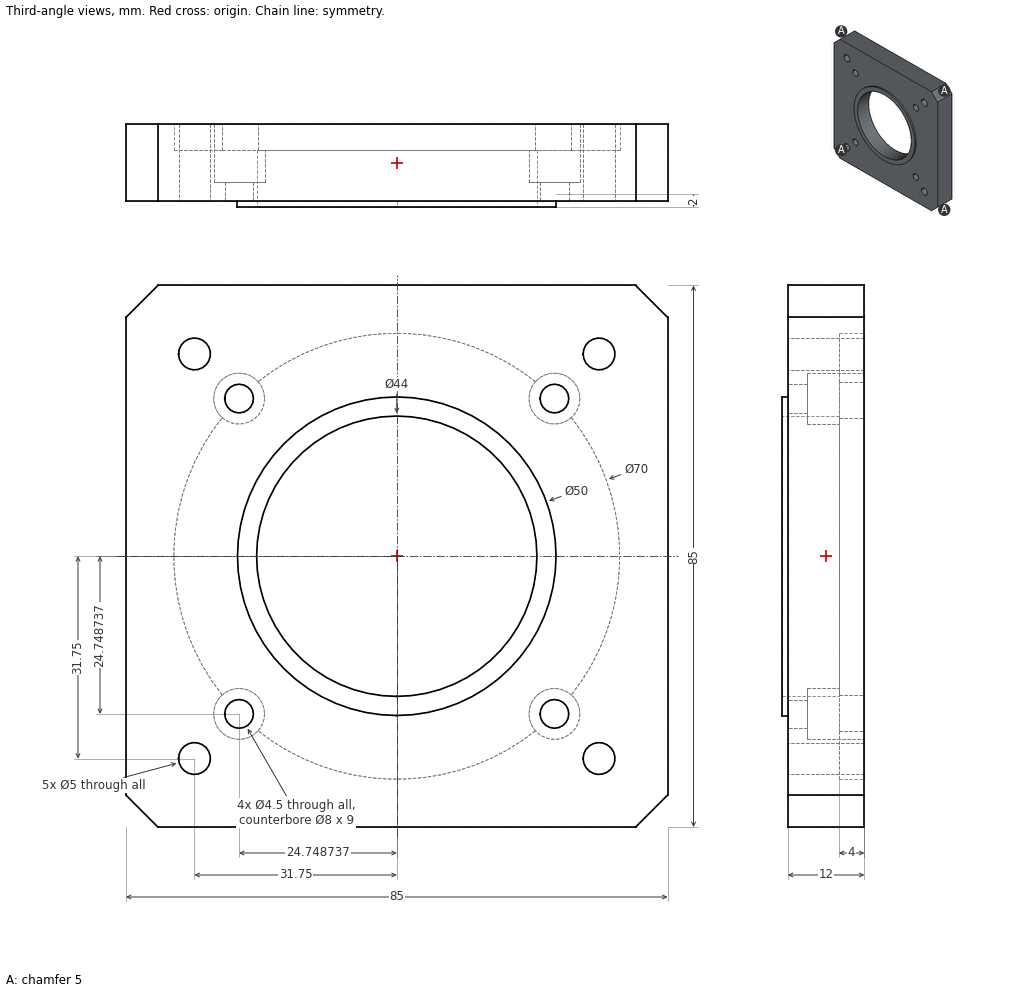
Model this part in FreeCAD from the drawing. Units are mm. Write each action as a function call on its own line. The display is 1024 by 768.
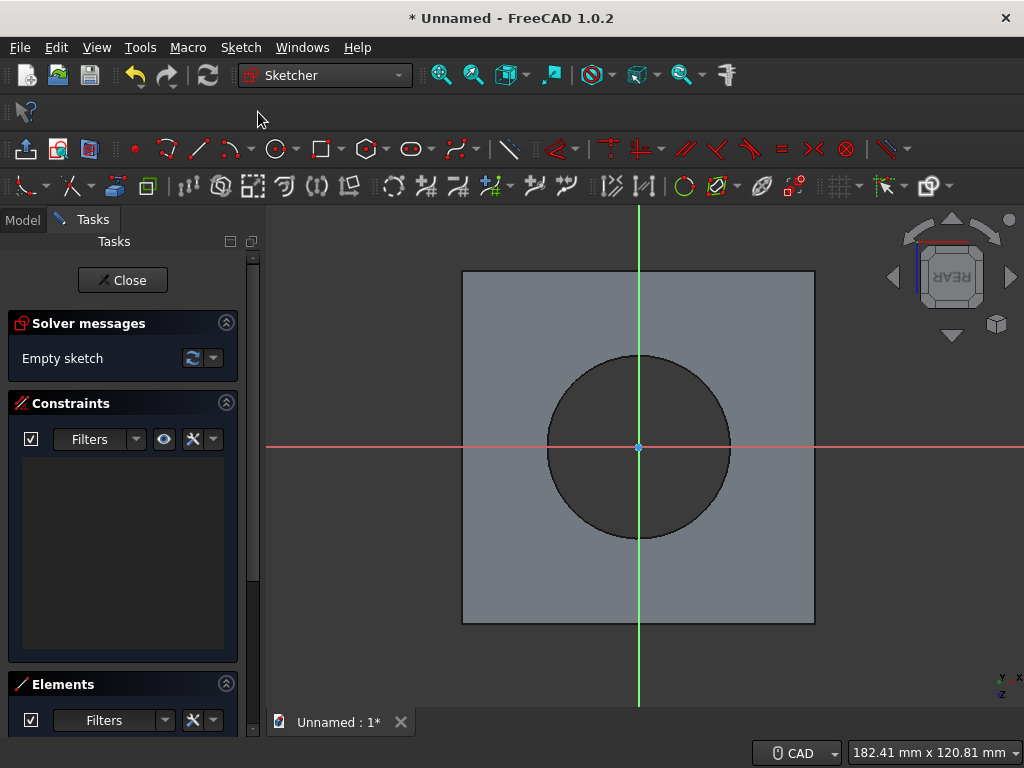
click(276, 150)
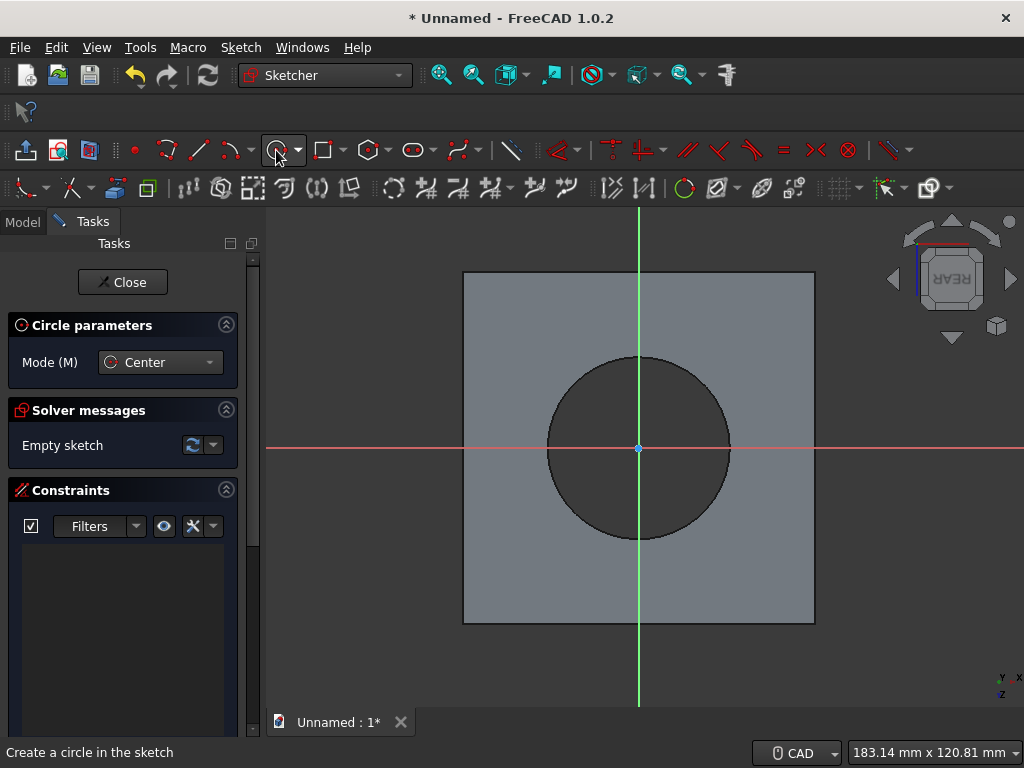
click(639, 448)
move(741, 346)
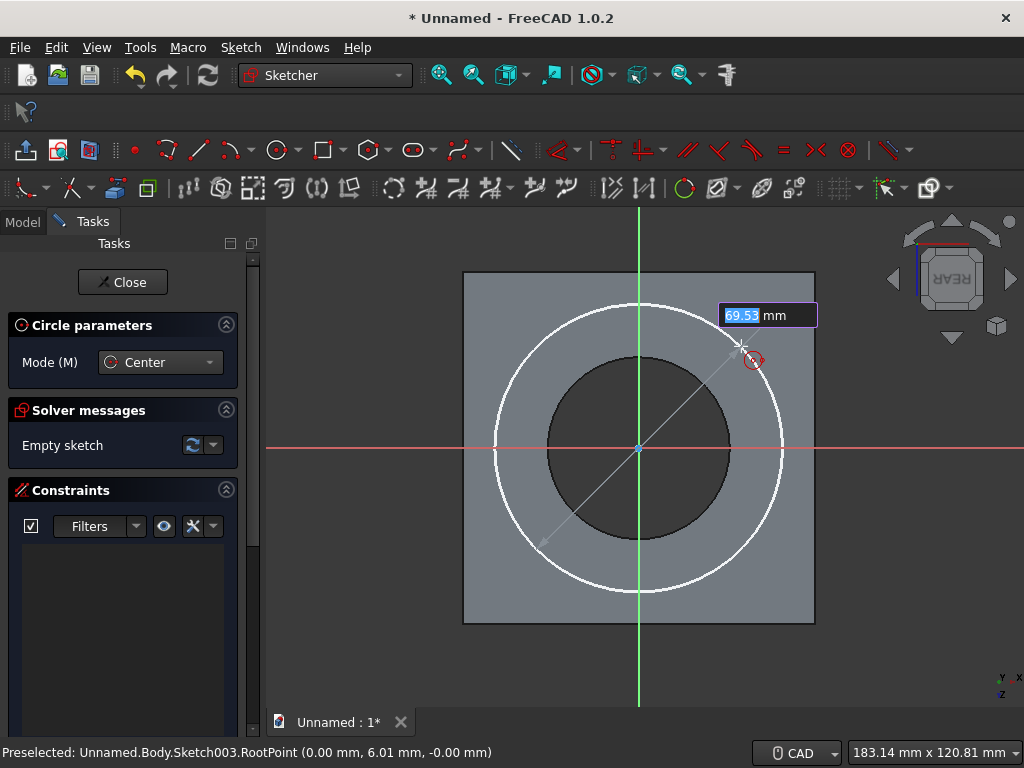
text(70)
key(Return)
key(Escape)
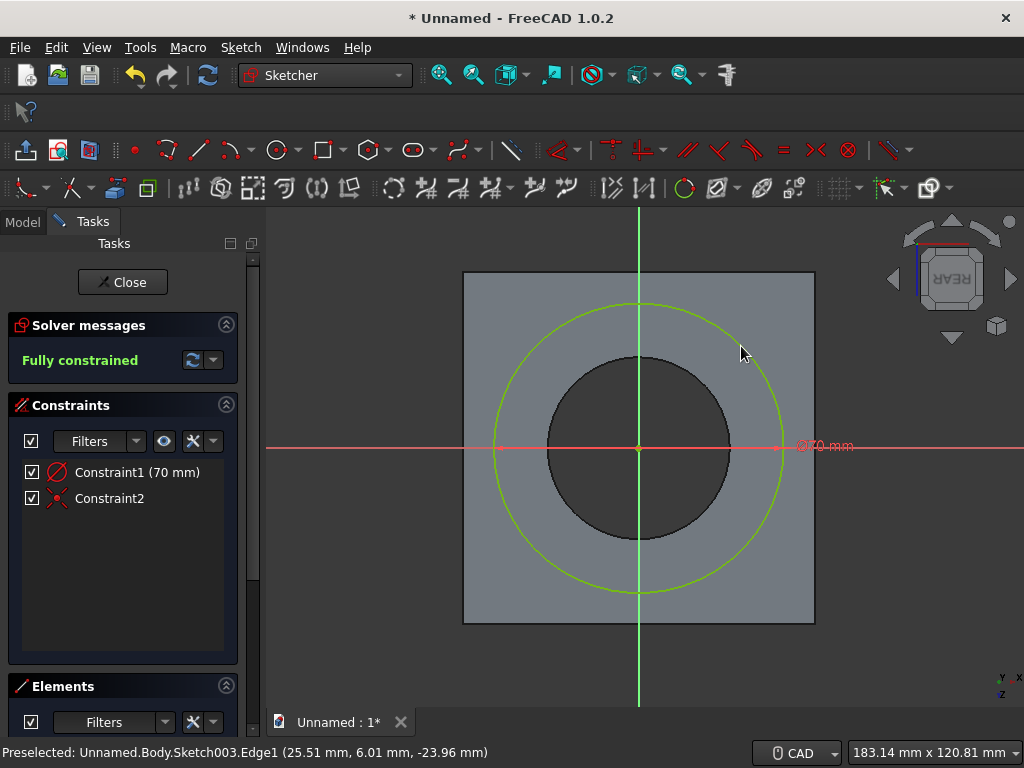
click(123, 282)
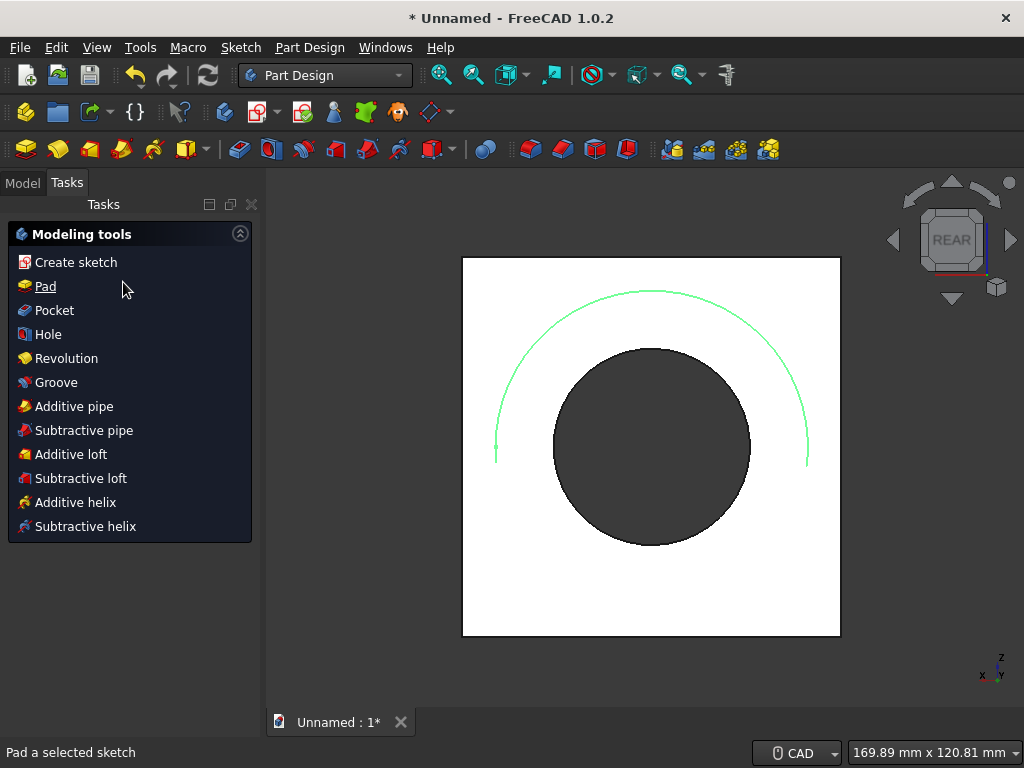
click(240, 150)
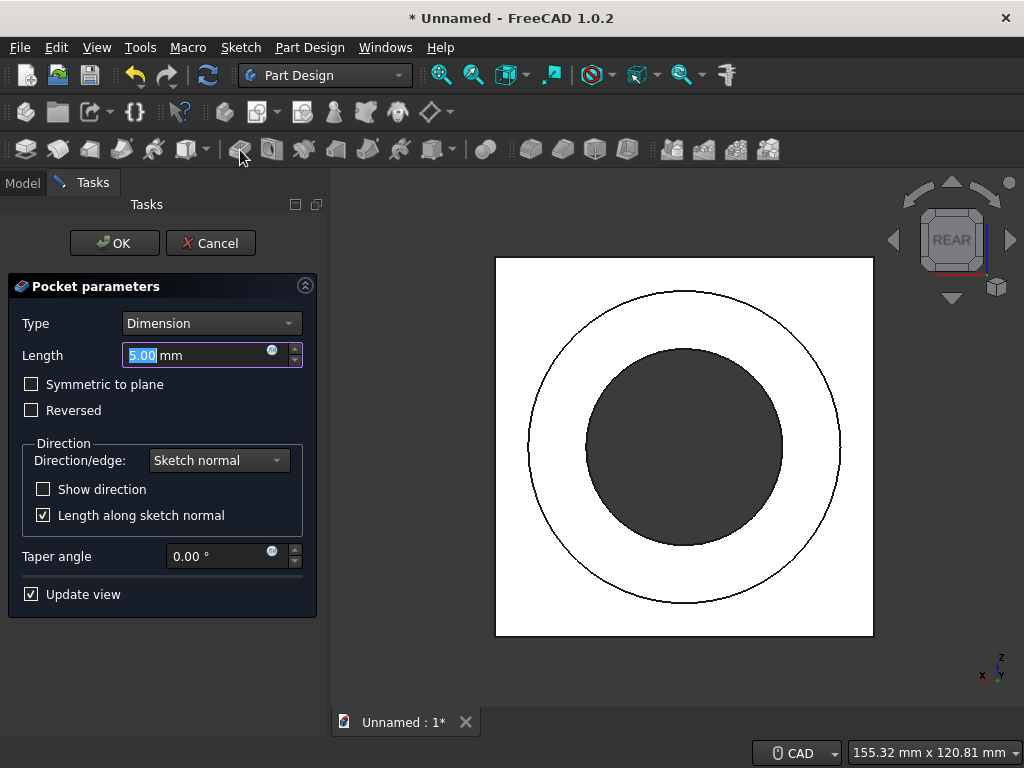
text(4)
key(Tab)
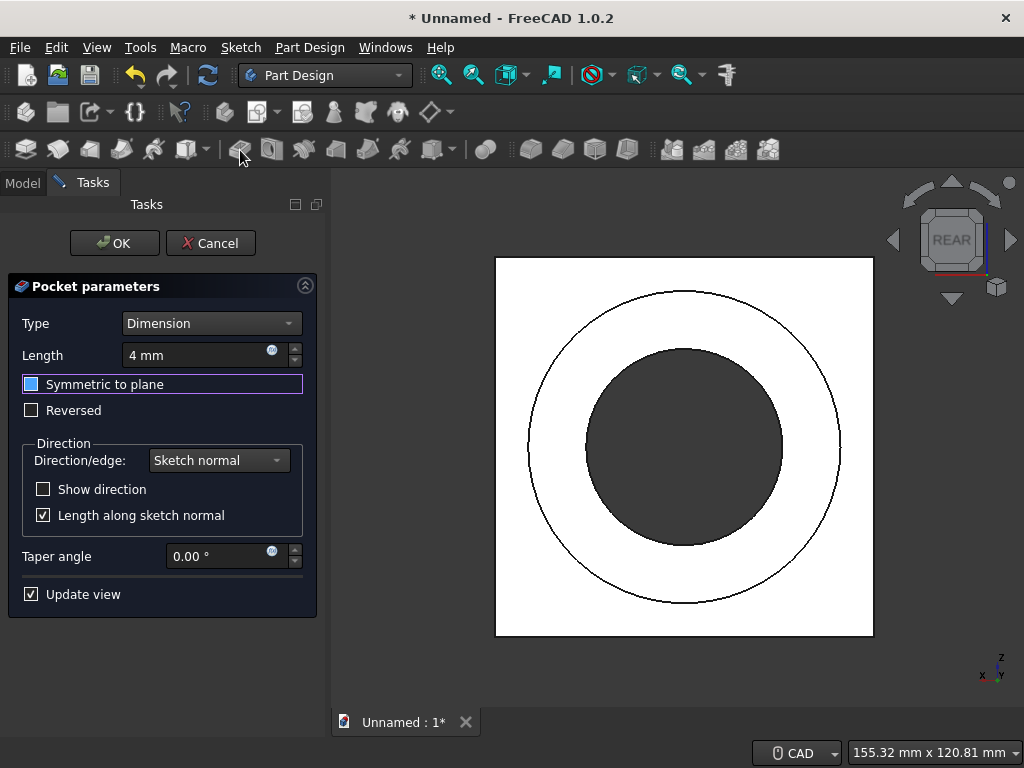
click(115, 243)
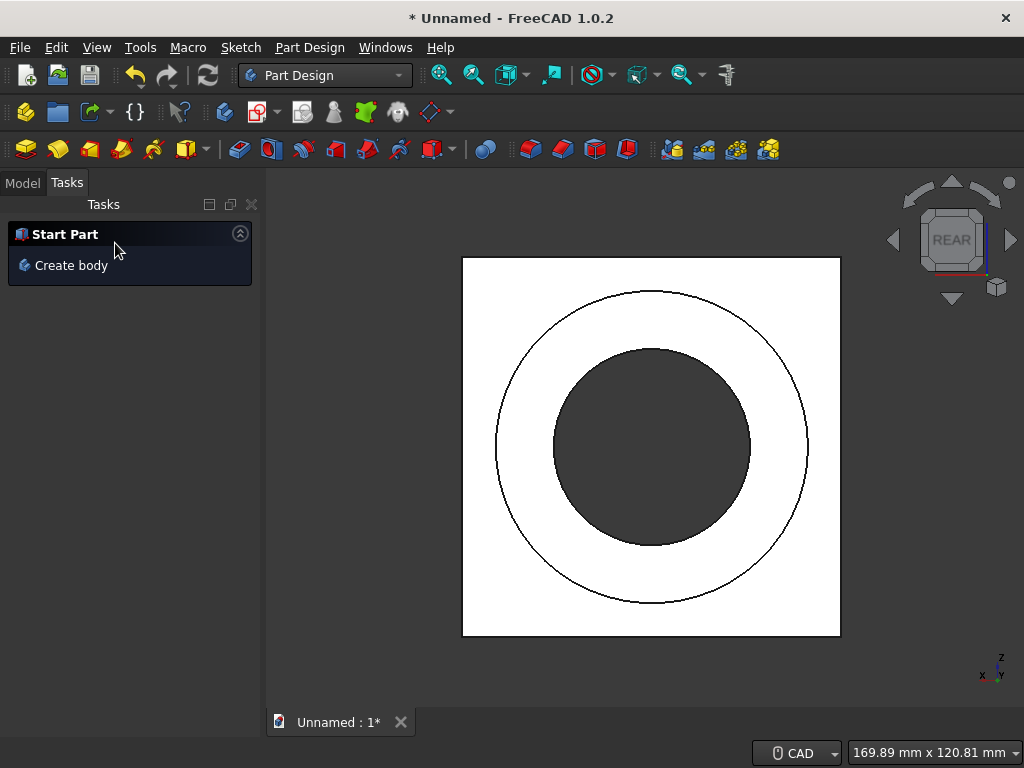
click(489, 284)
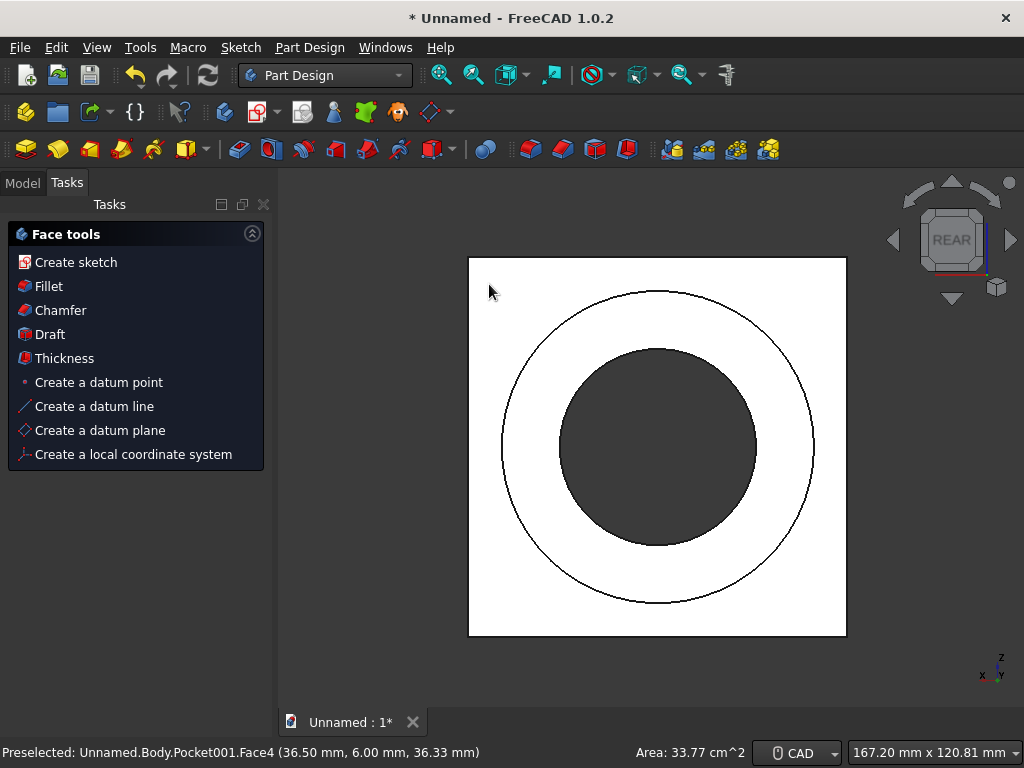
click(258, 112)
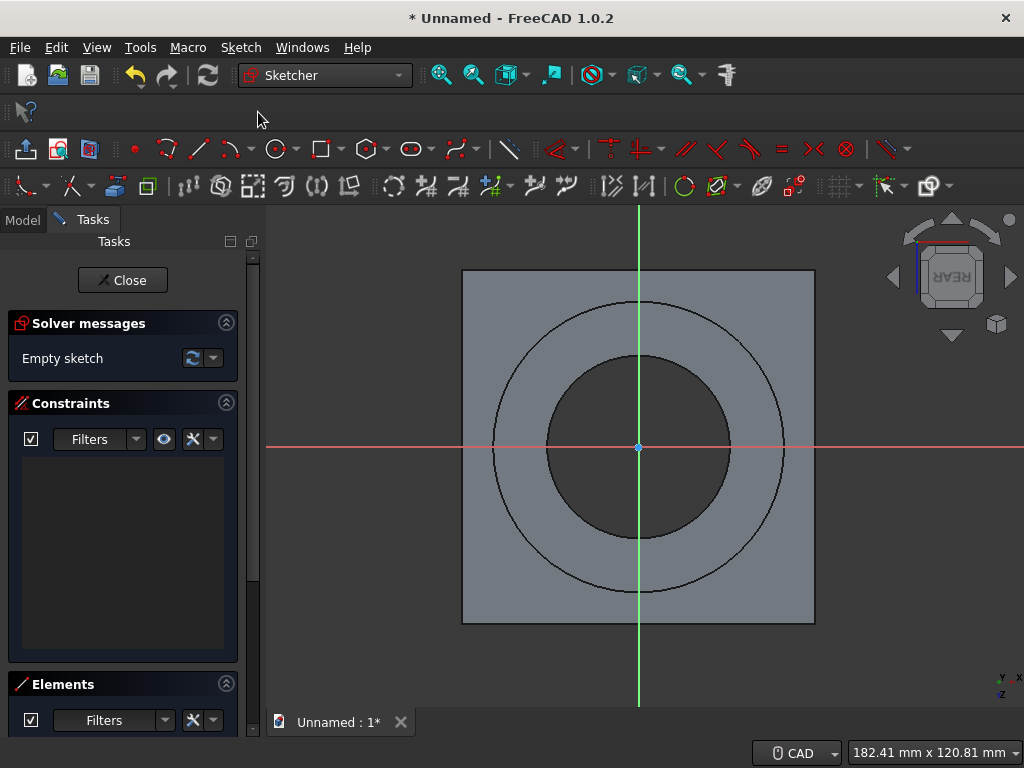
click(276, 150)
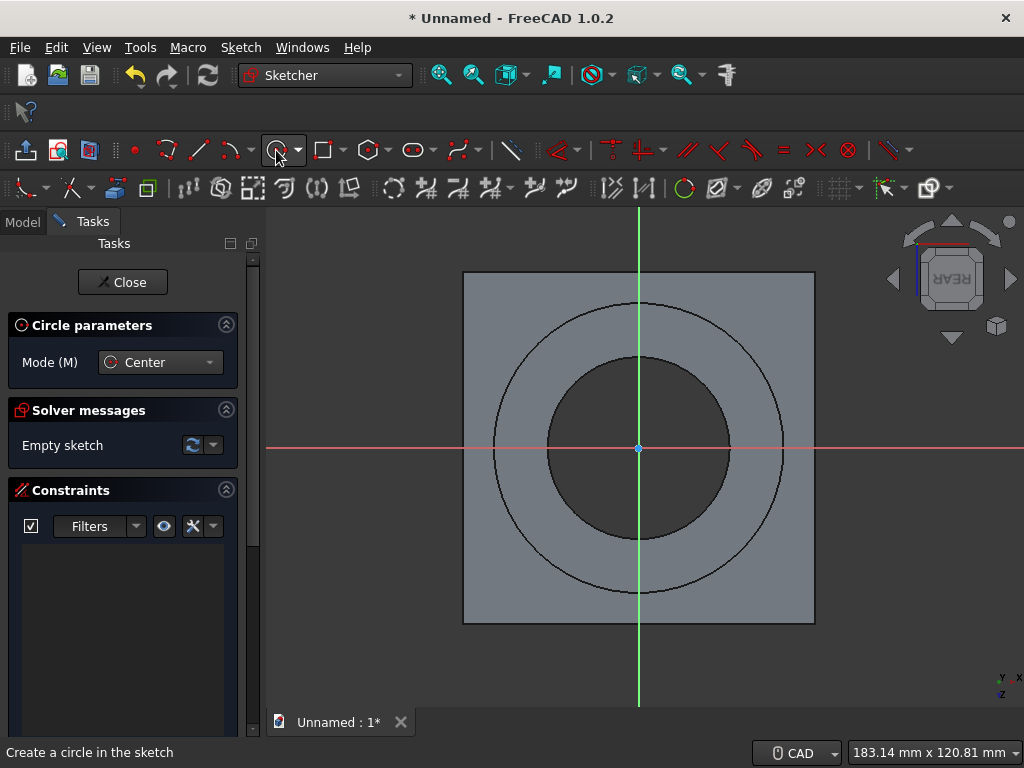
scroll(507, 317, up, 4)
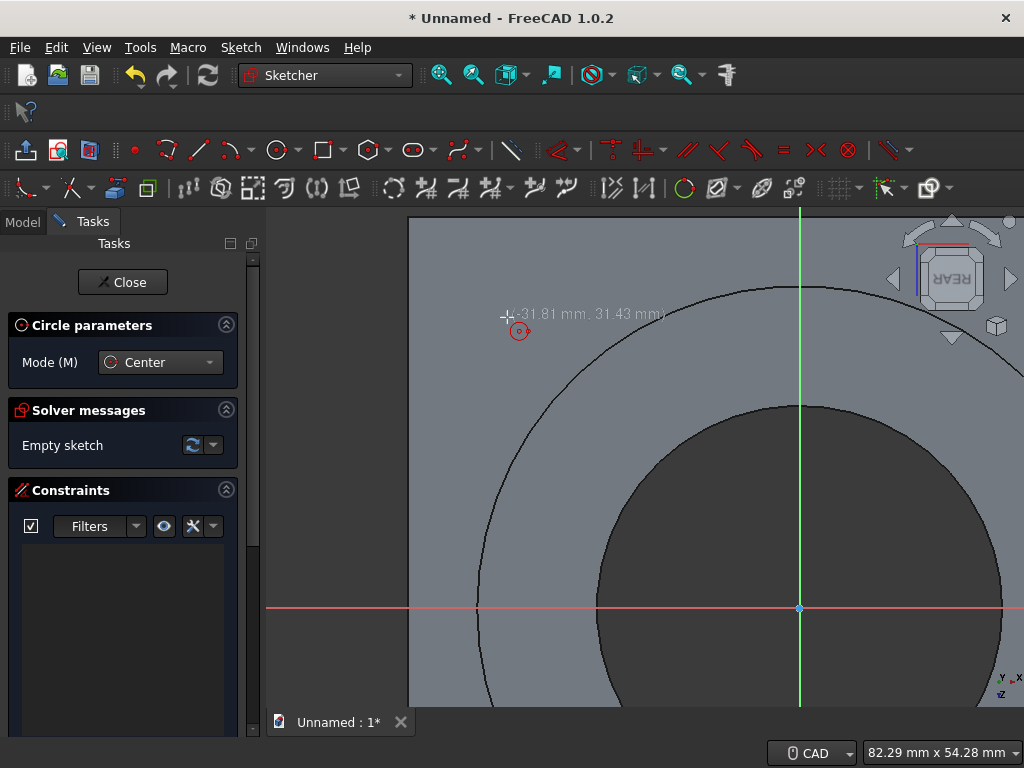
click(507, 316)
move(523, 300)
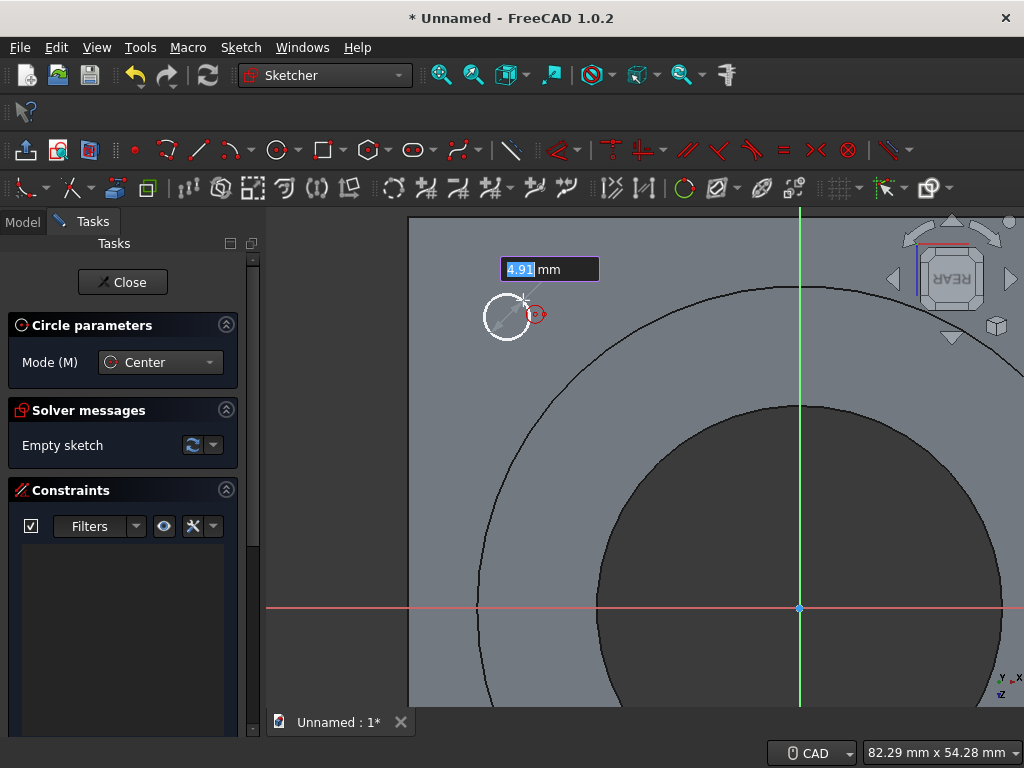
text(5)
key(Return)